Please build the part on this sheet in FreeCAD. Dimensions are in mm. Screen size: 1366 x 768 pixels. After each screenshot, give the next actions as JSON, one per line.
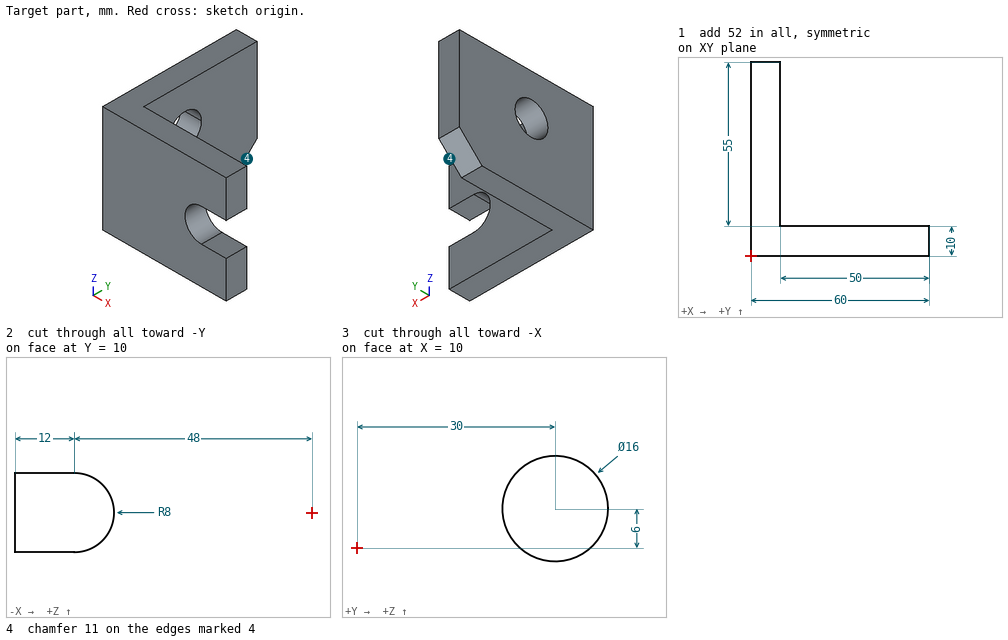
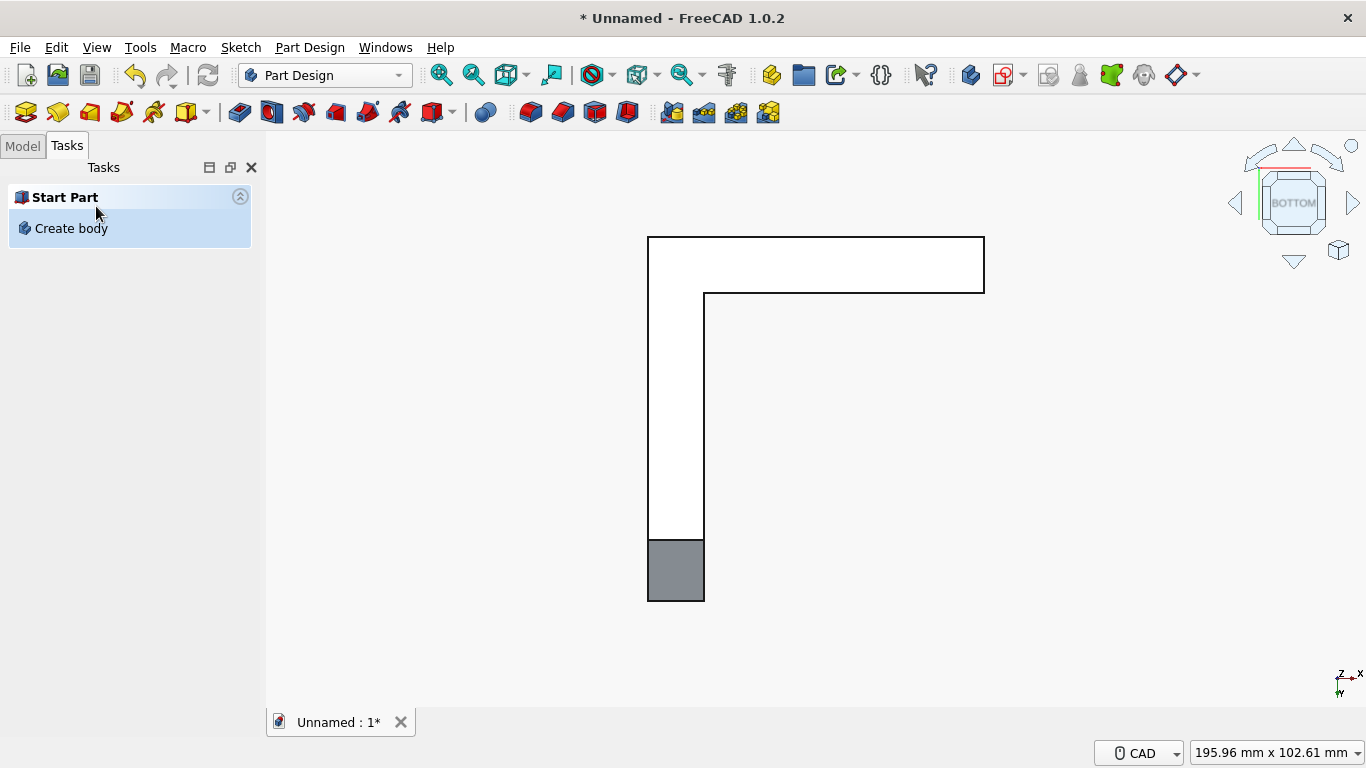
{"action": "key", "text": "0"}